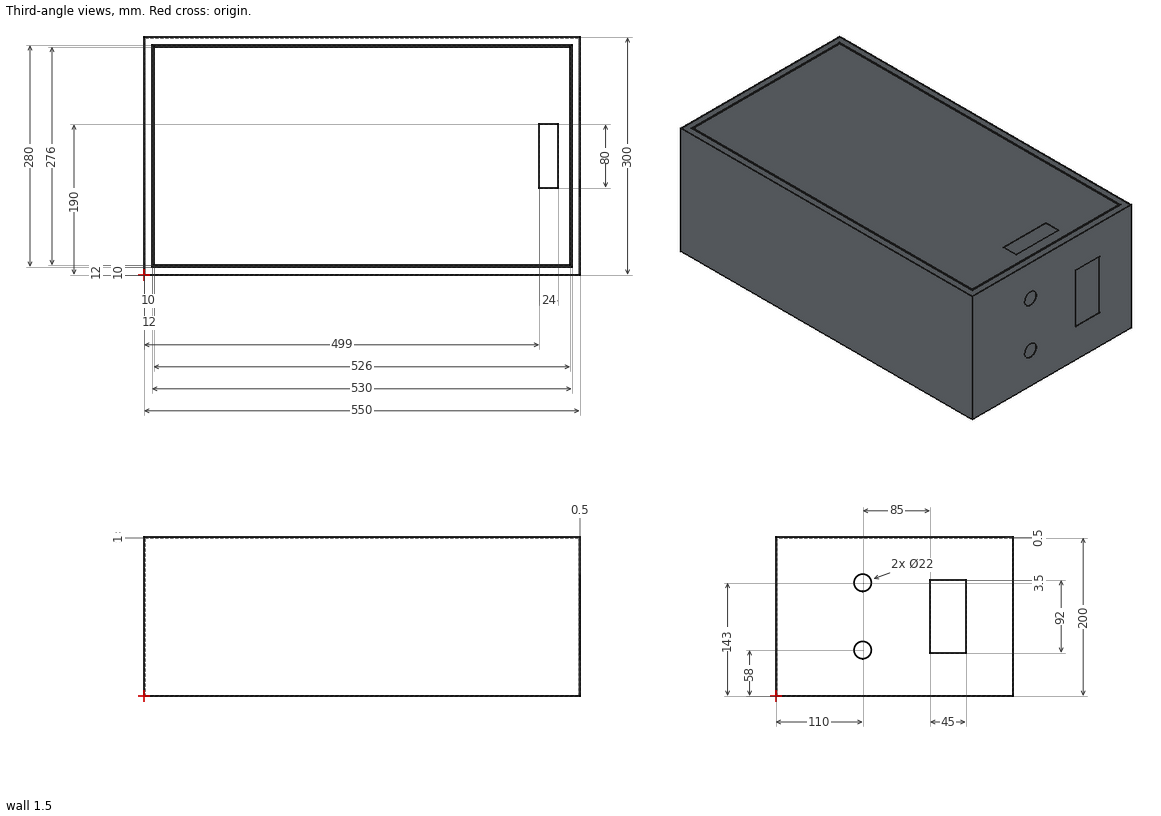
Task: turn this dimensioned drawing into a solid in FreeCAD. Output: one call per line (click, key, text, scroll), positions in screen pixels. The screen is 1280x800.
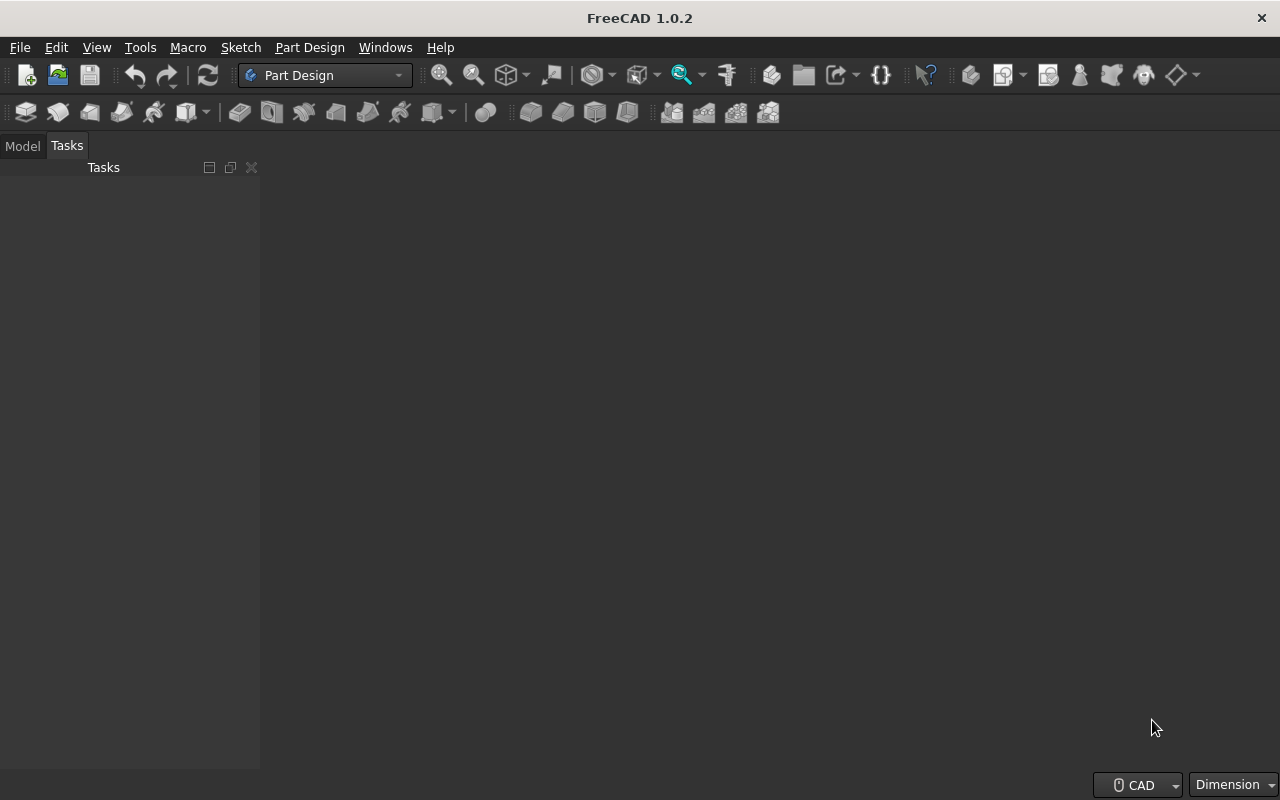
click(26, 76)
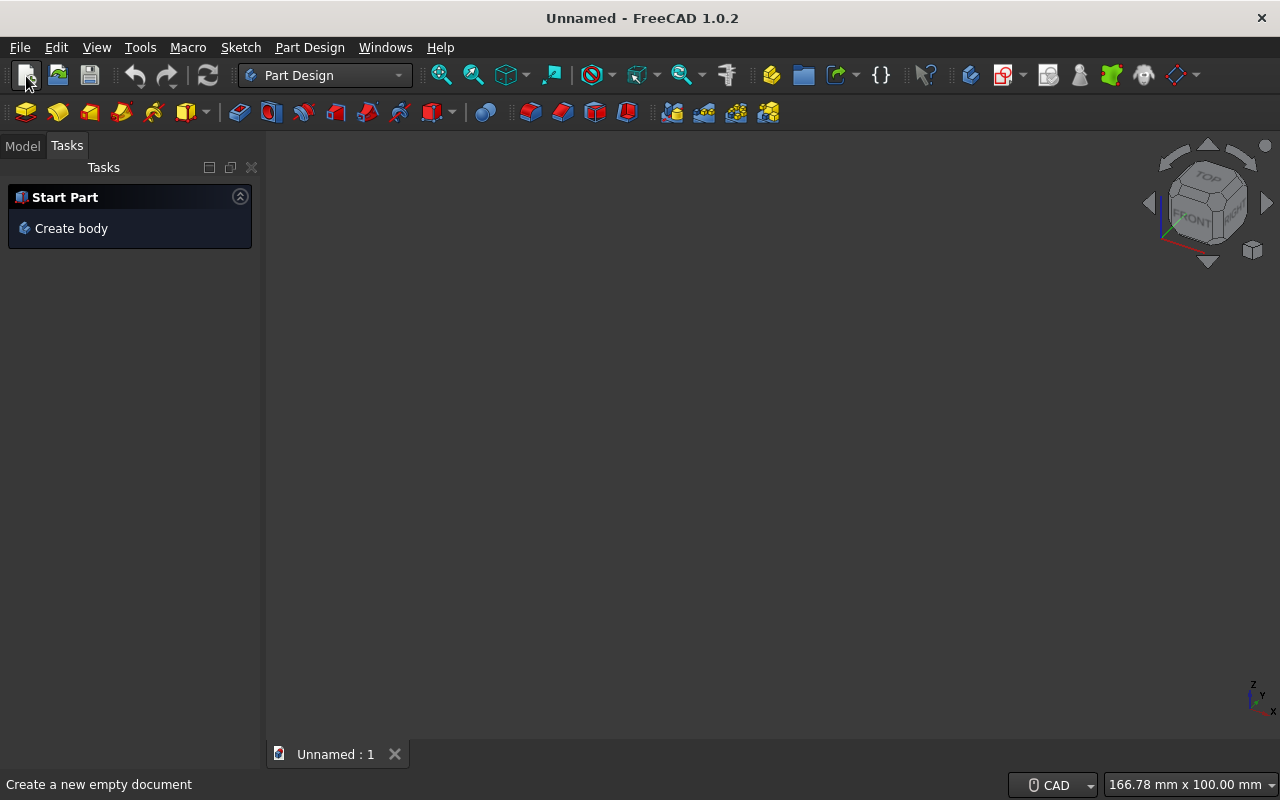
click(1004, 76)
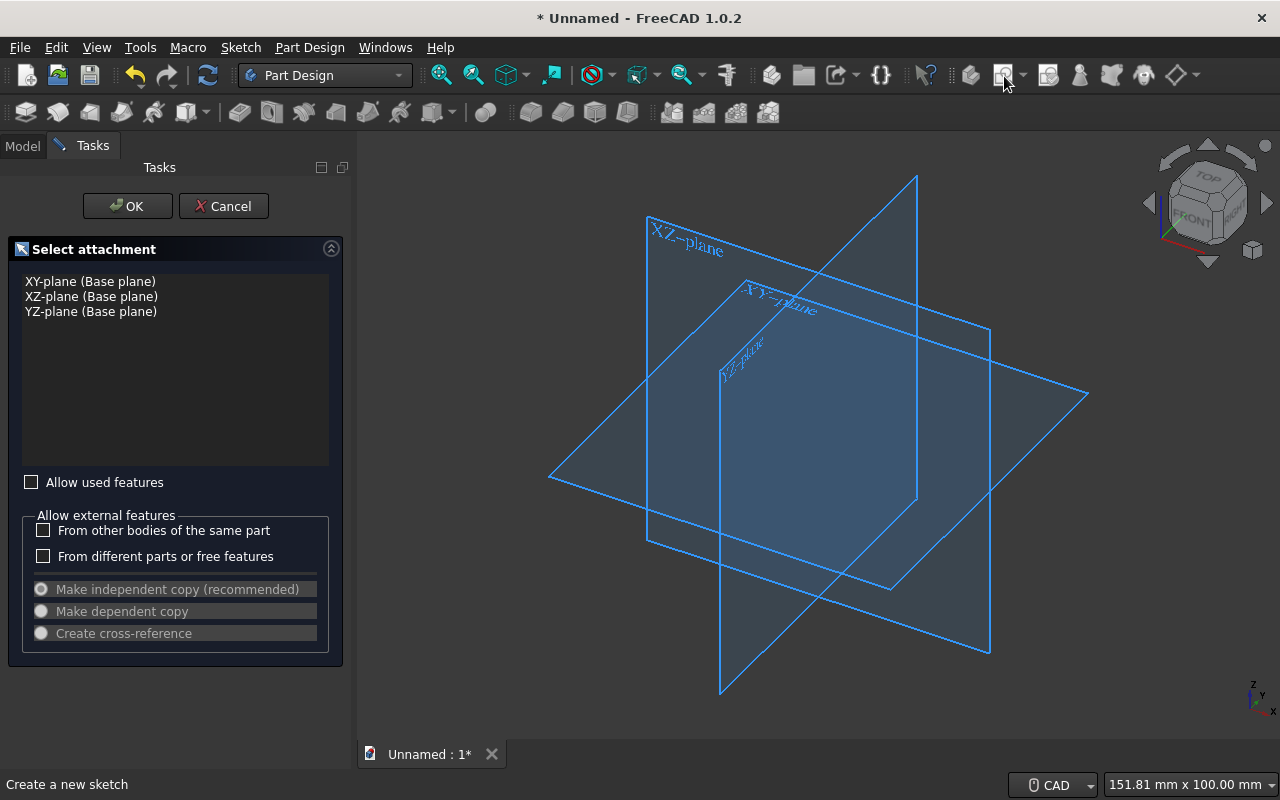
click(82, 282)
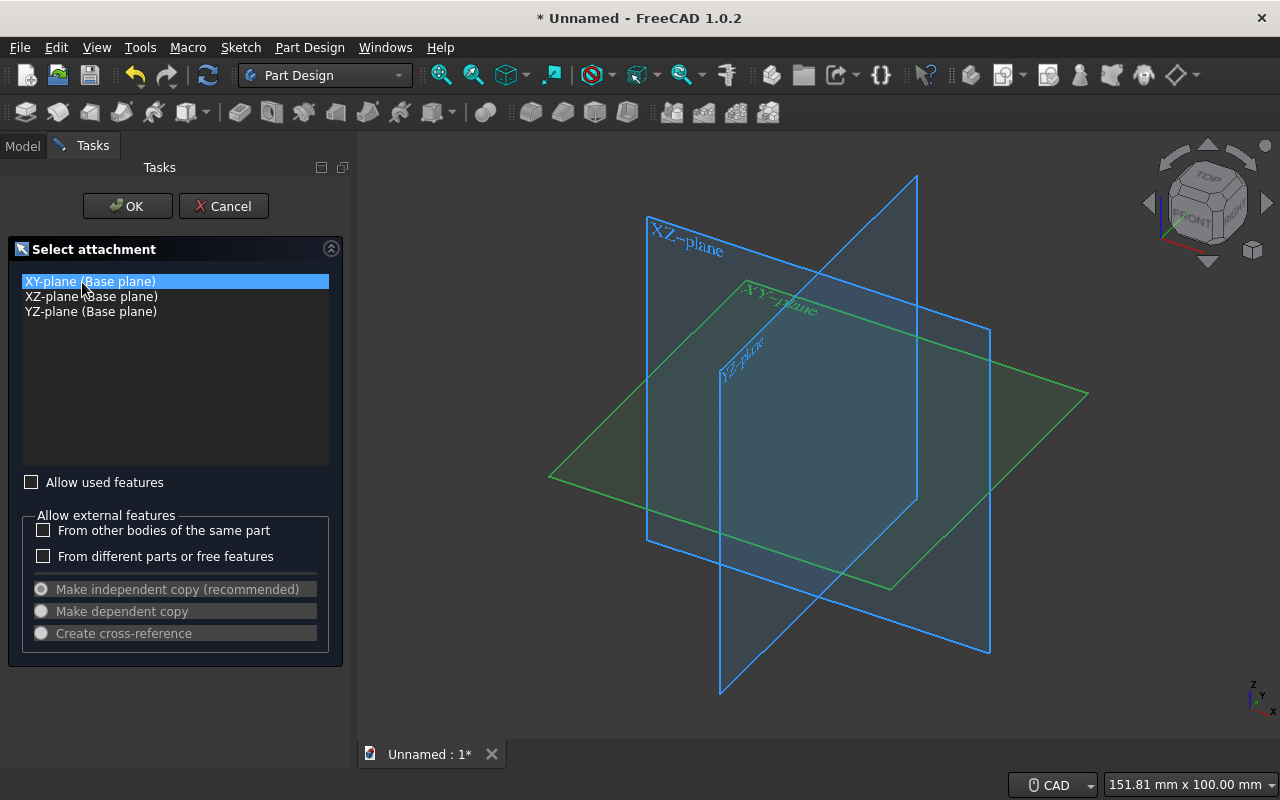
click(128, 206)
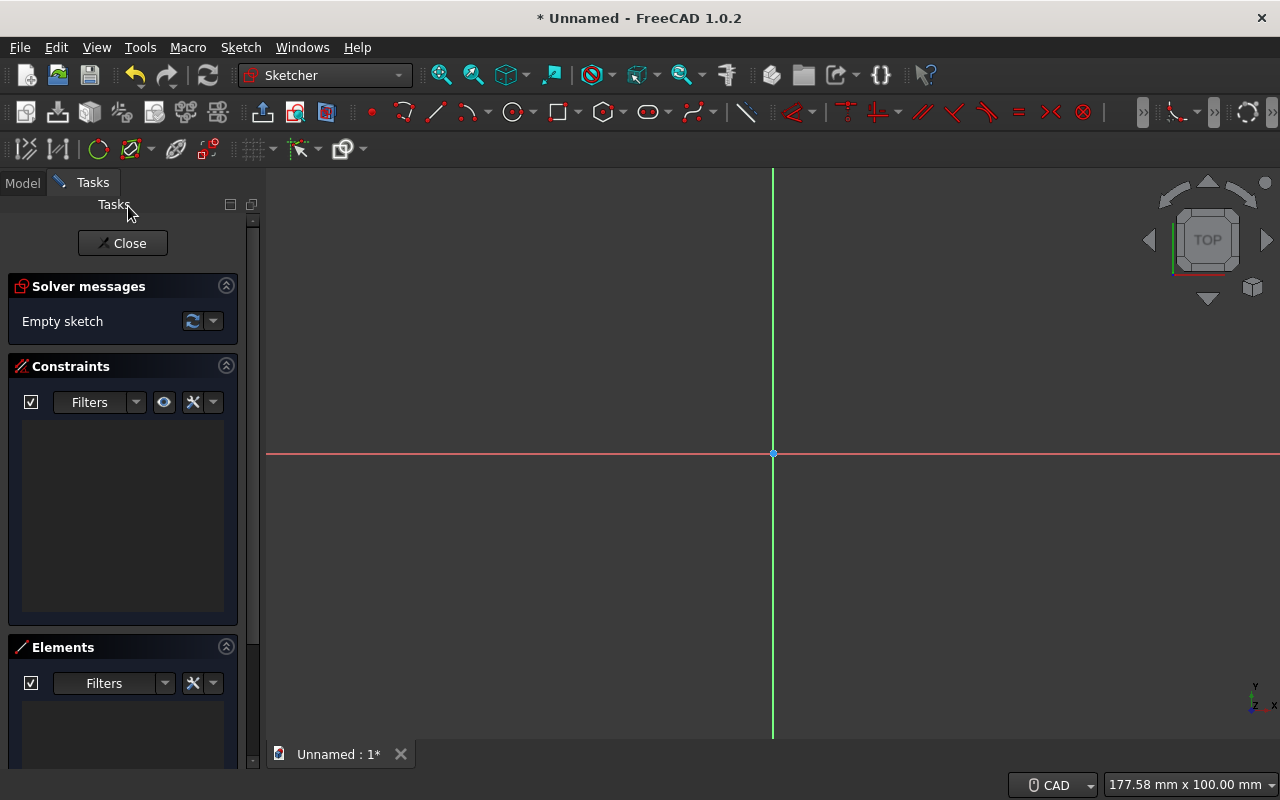
scroll(294, 670, down, 8)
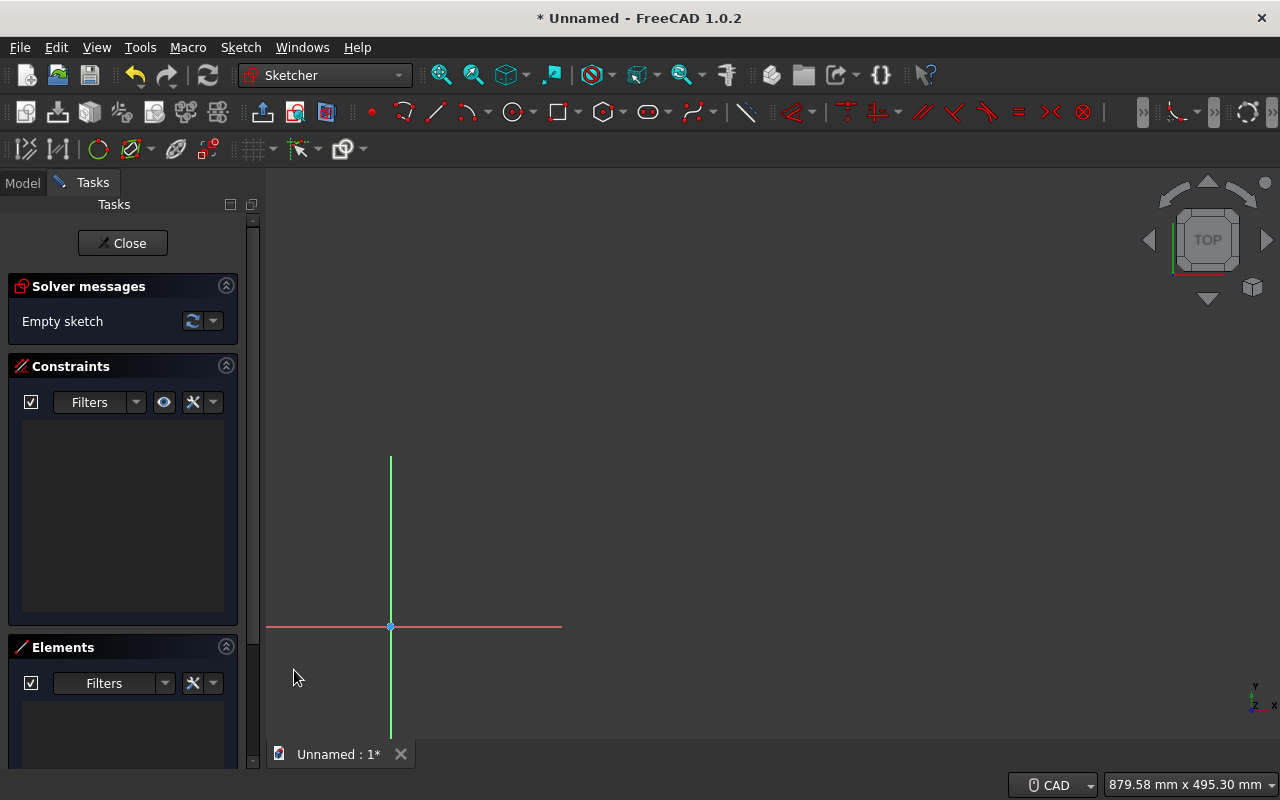
click(558, 112)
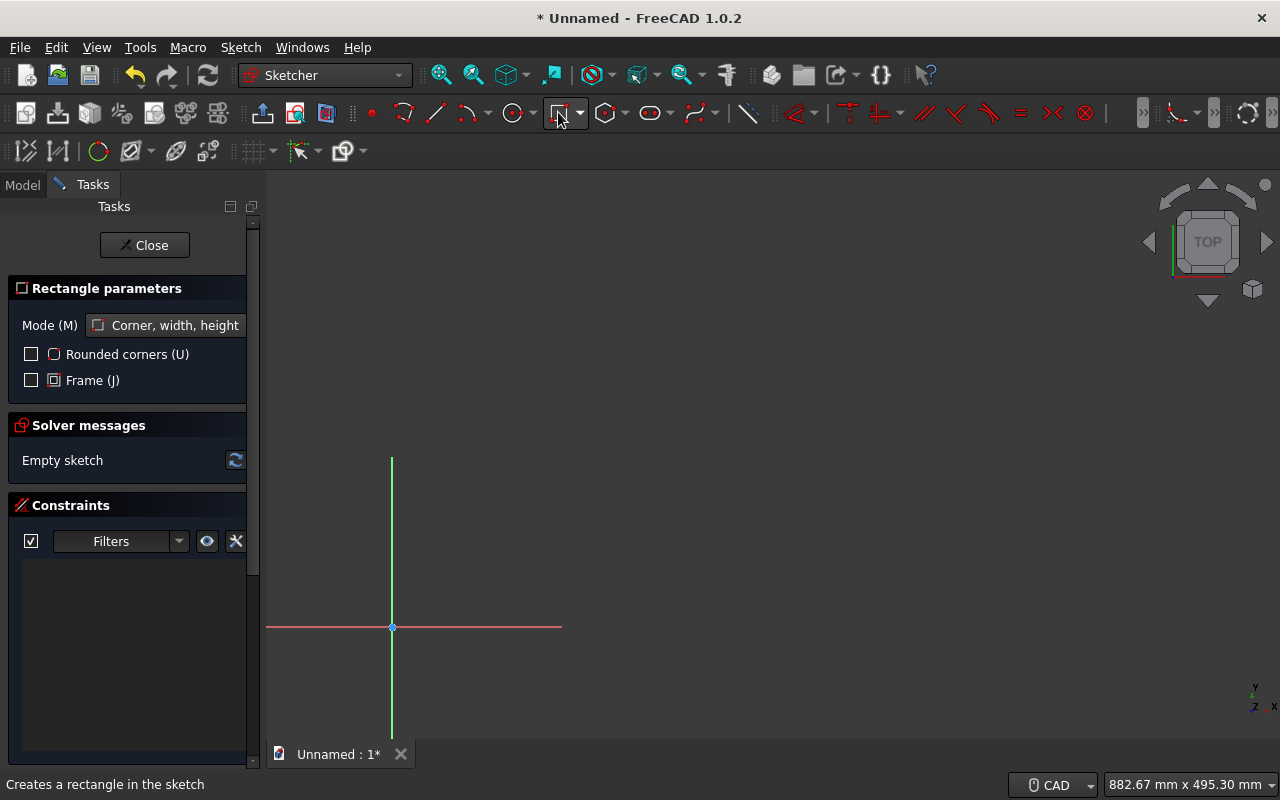
click(392, 627)
move(1024, 283)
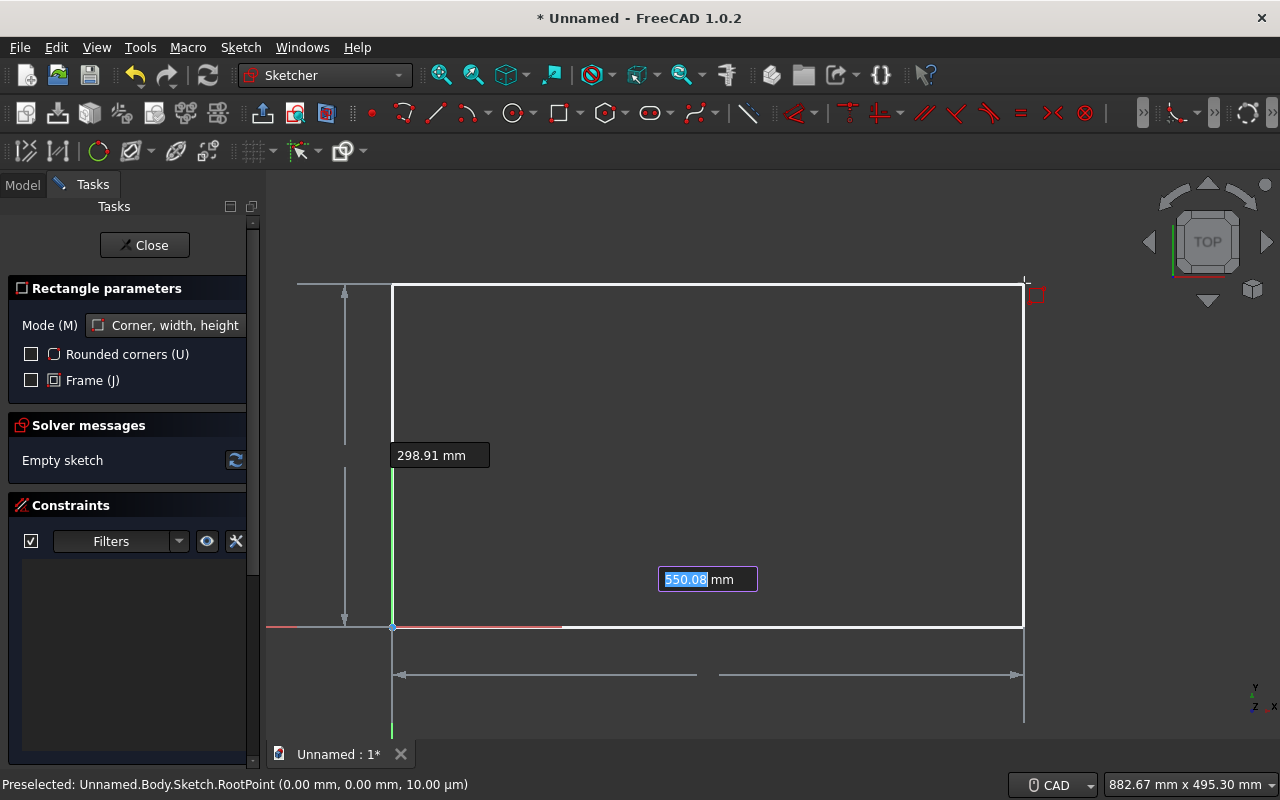
text(550)
key(Tab)
text(300)
key(Return)
key(Escape)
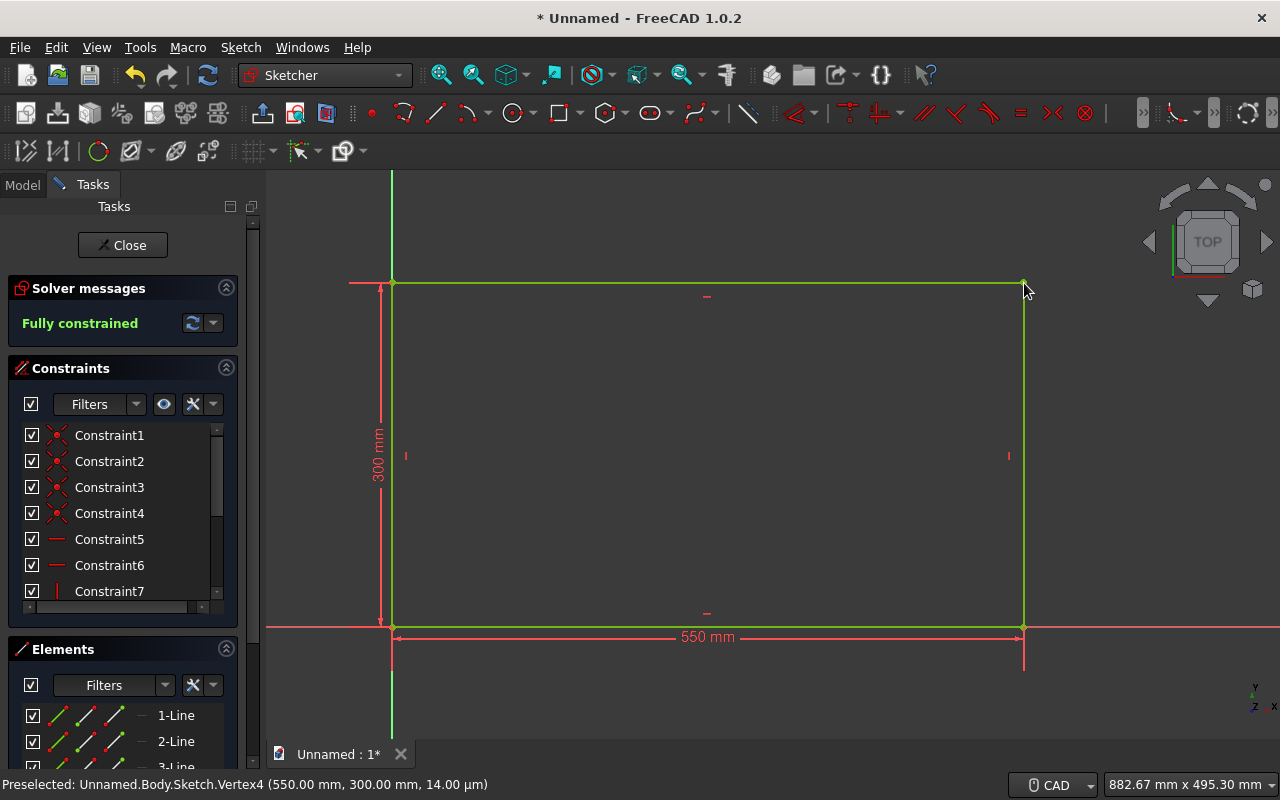
click(123, 245)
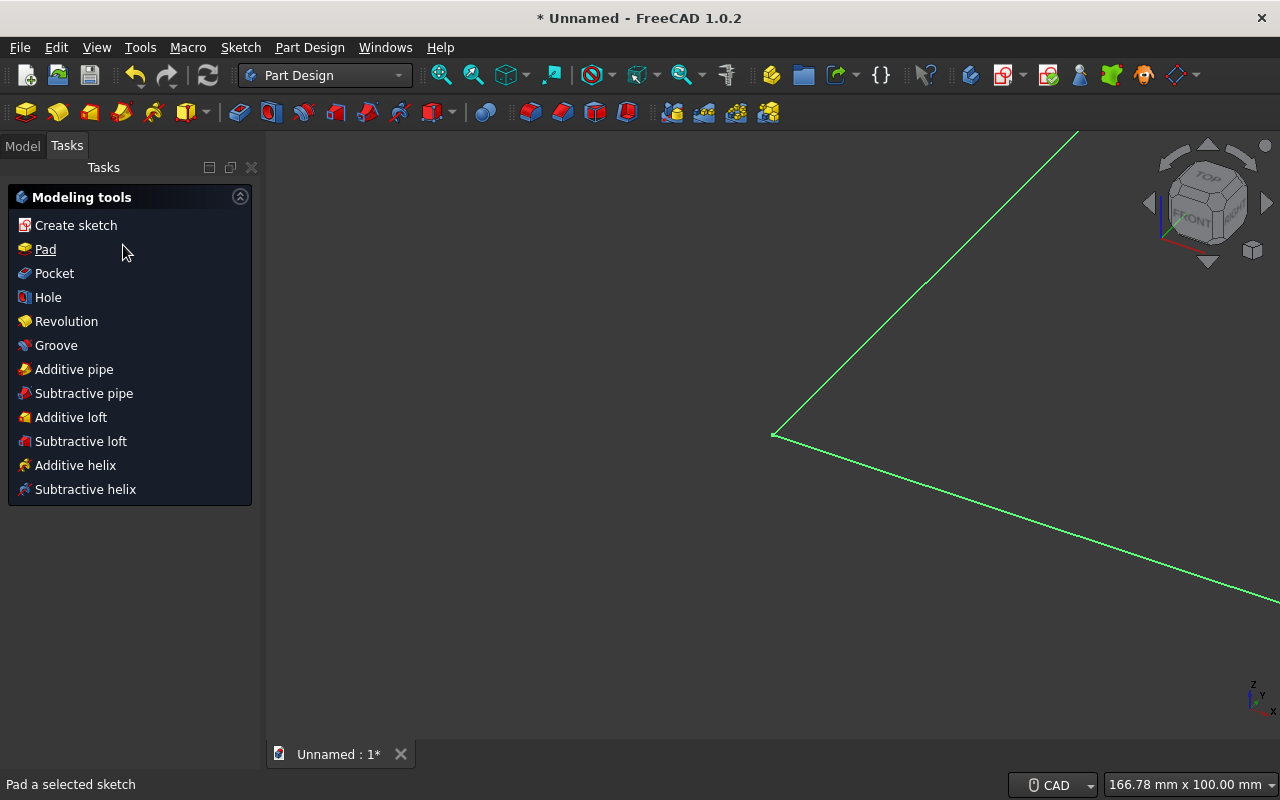
click(26, 112)